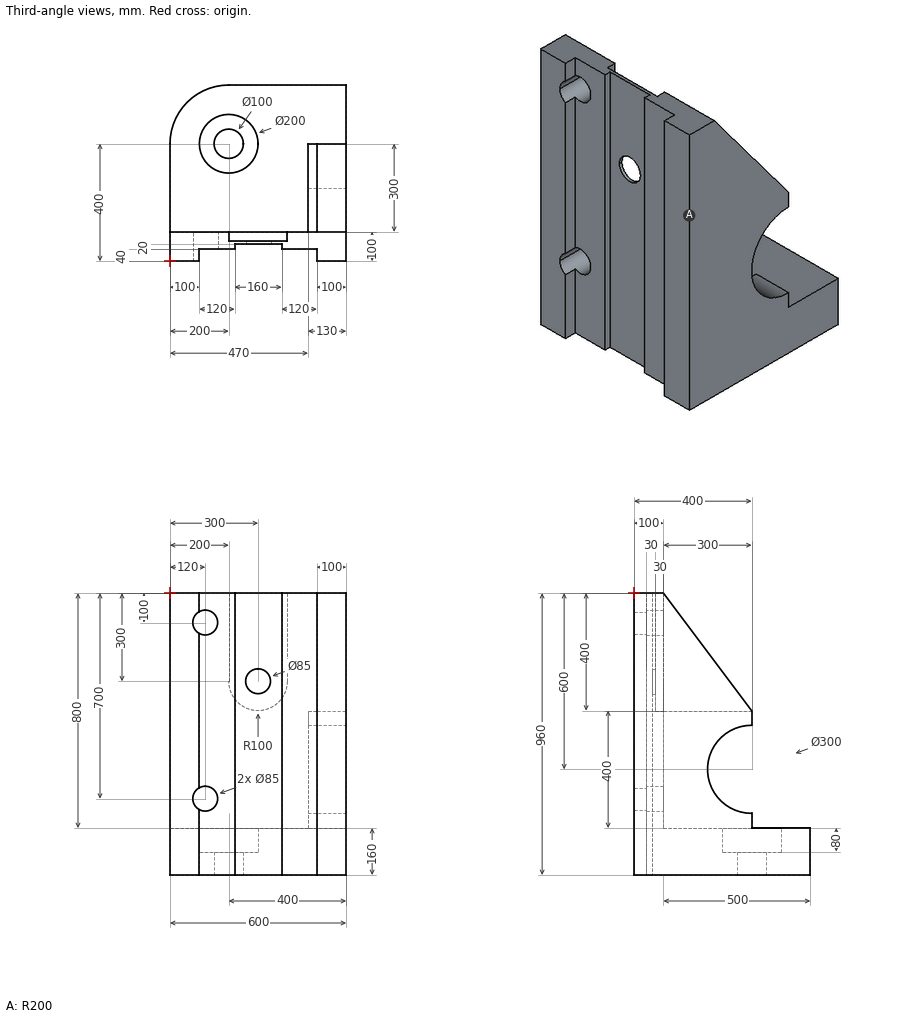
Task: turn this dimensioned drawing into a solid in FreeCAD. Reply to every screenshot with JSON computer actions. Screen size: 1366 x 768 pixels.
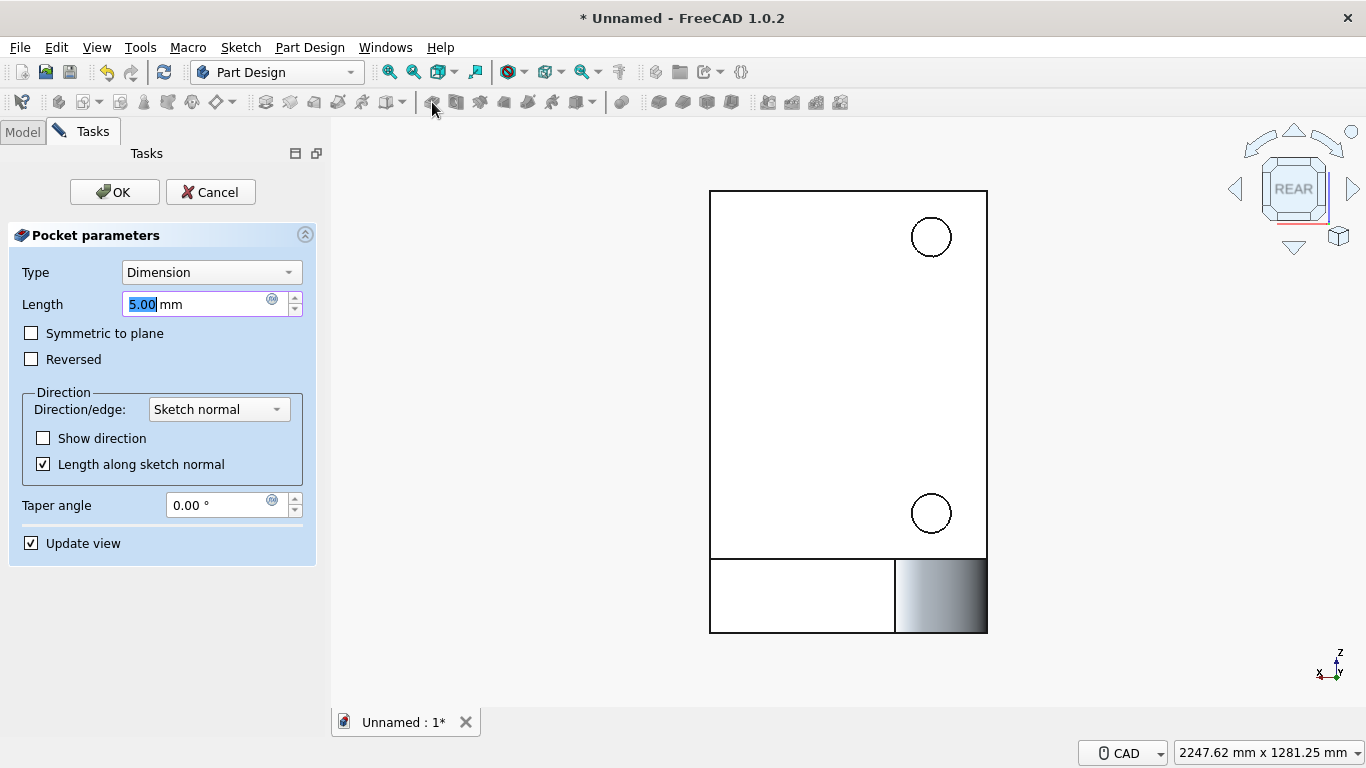
{"action": "left_click", "coordinate": [212, 272]}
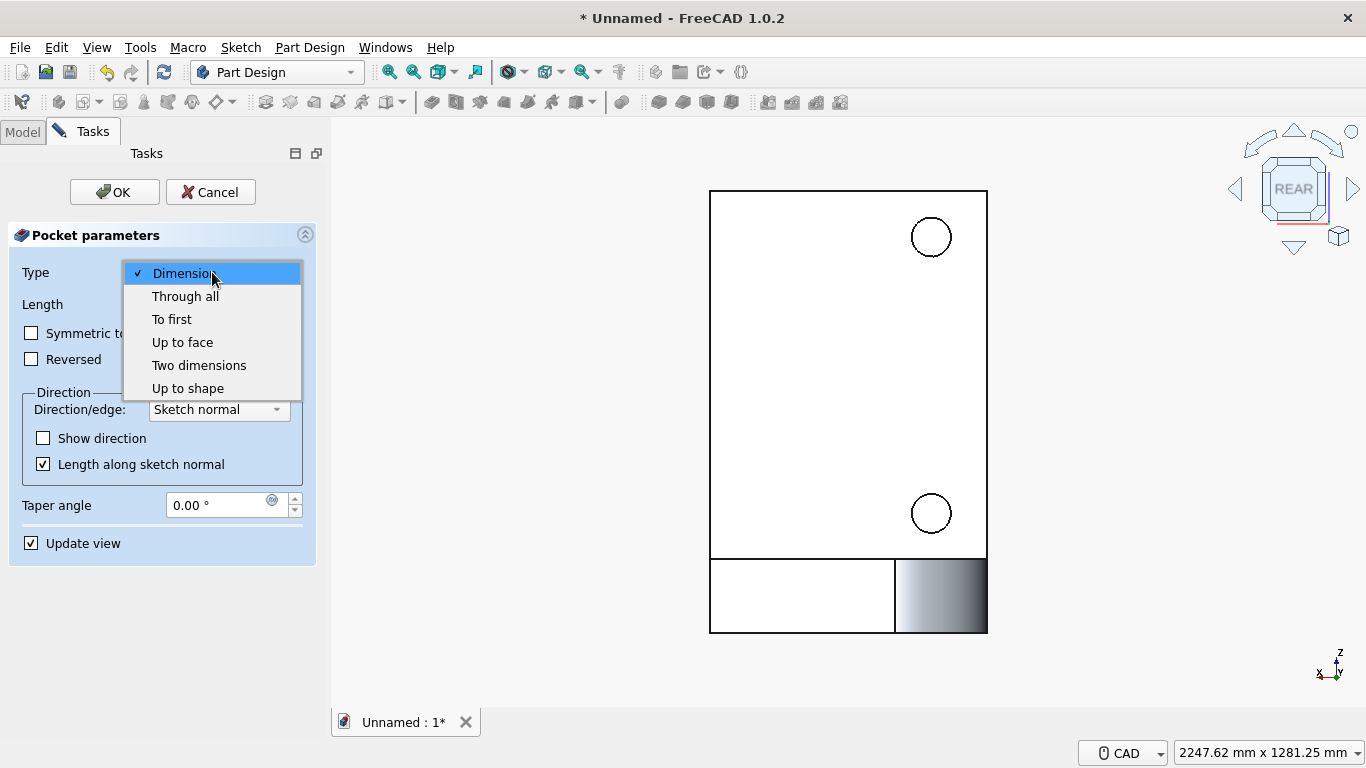
{"action": "left_click", "coordinate": [212, 296]}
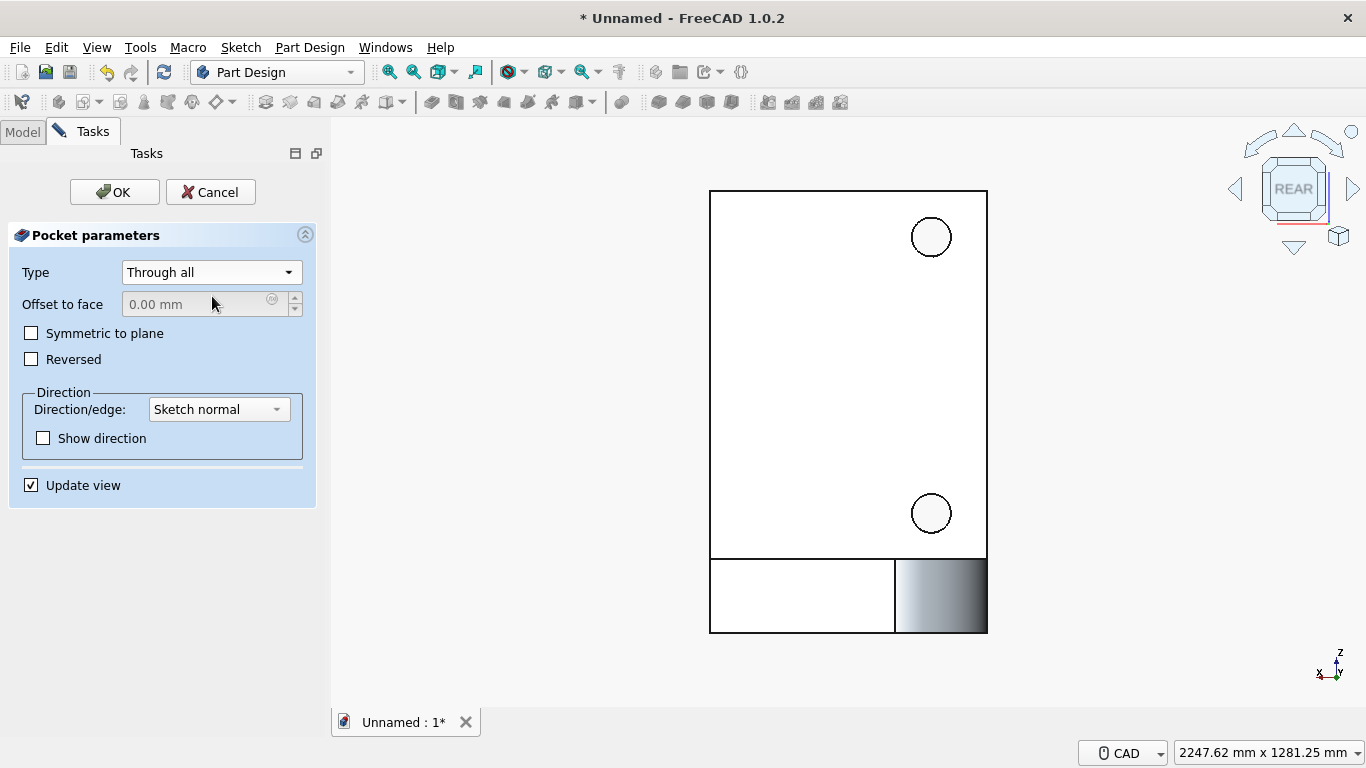
{"action": "left_click", "coordinate": [115, 192]}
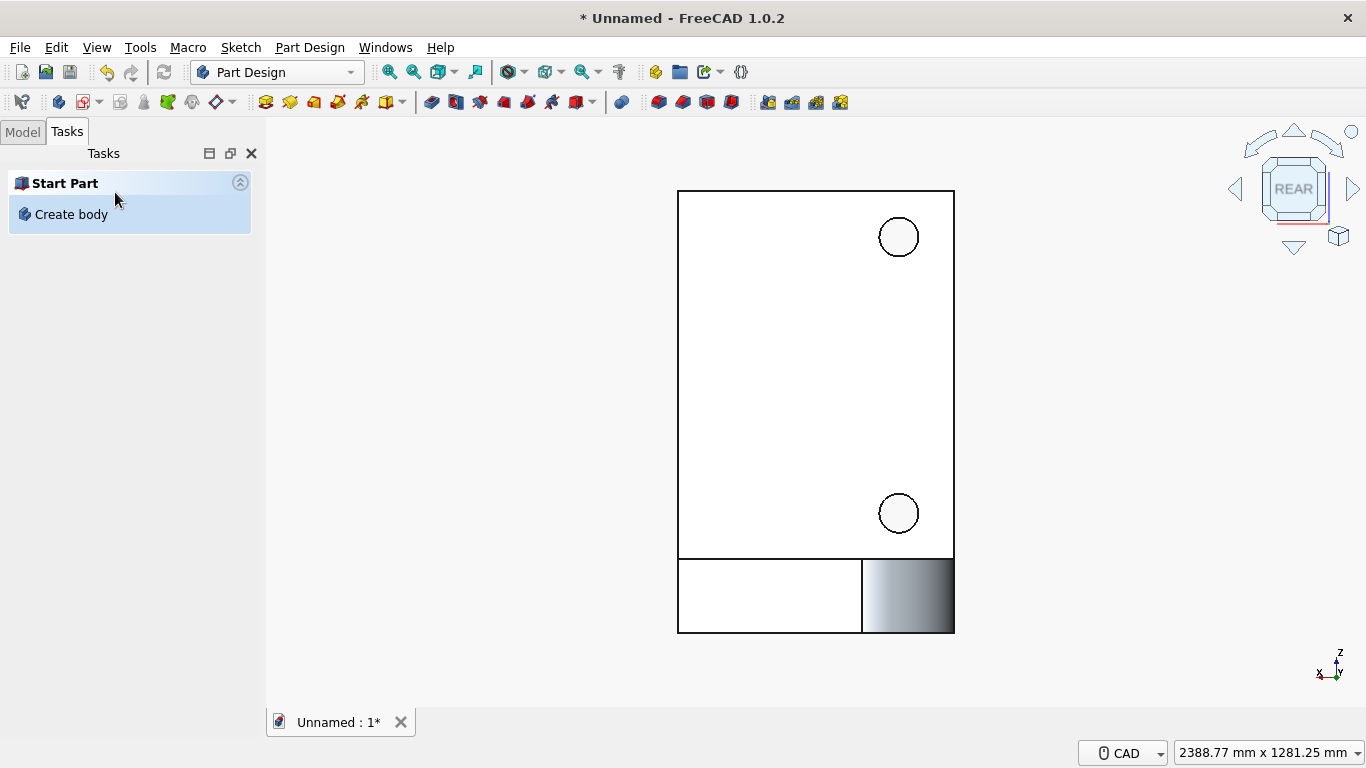
{"action": "left_click", "coordinate": [816, 374]}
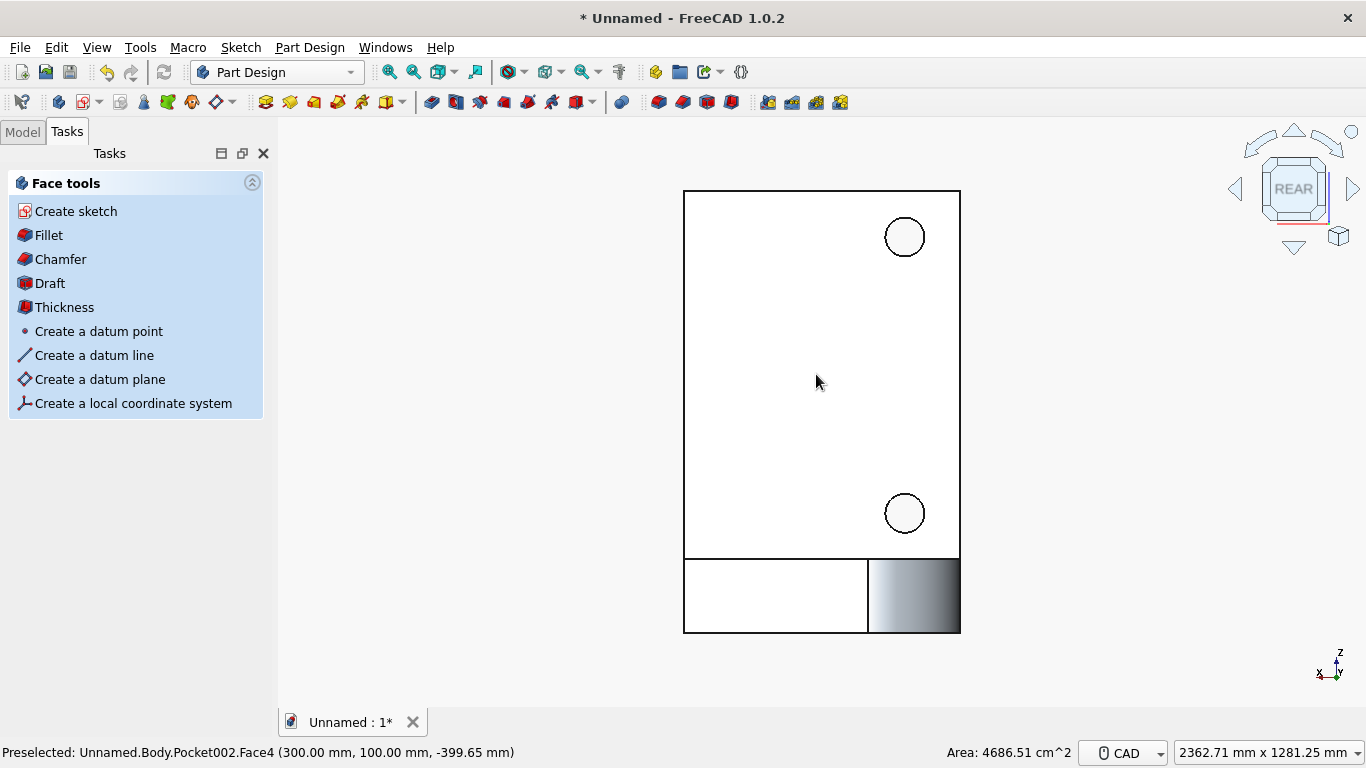
{"action": "left_click", "coordinate": [84, 102]}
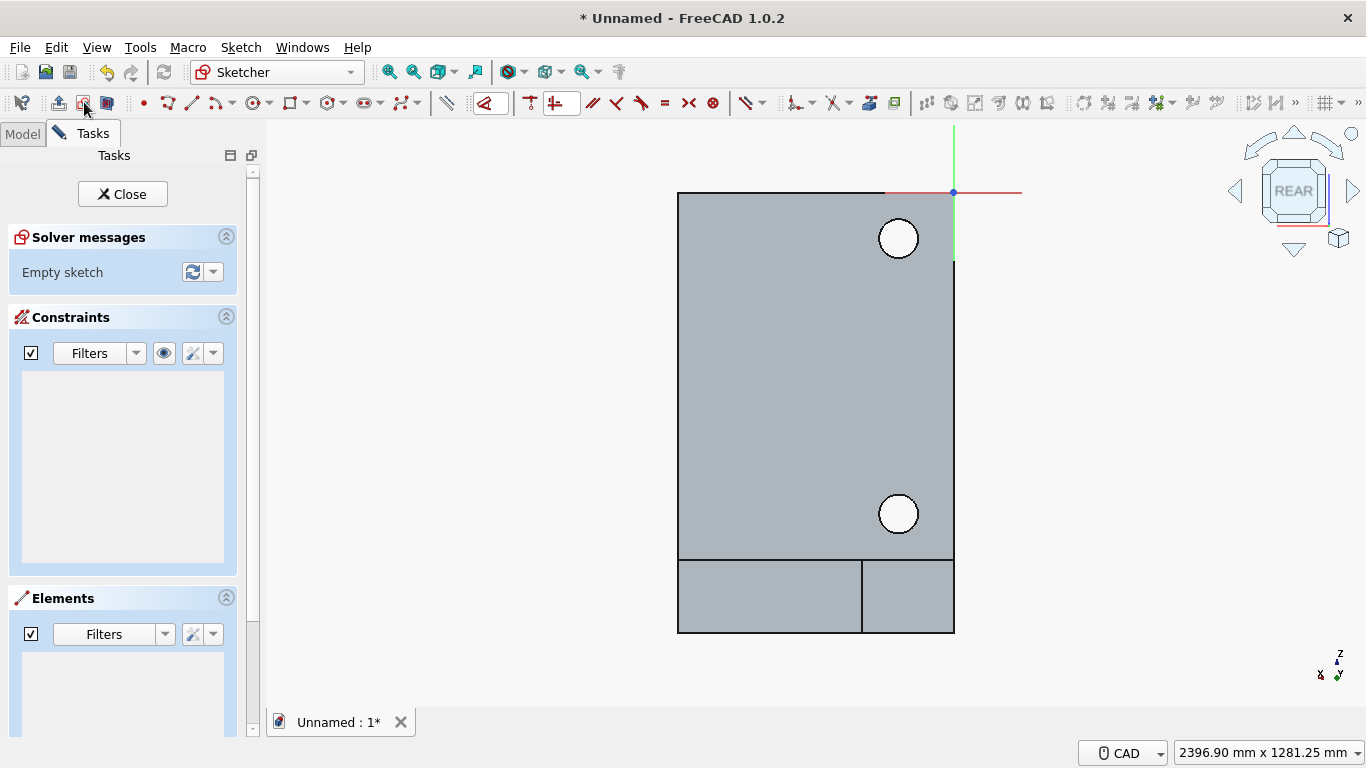
{"action": "scroll", "coordinate": [955, 180], "scroll_direction": "up", "scroll_amount": 4}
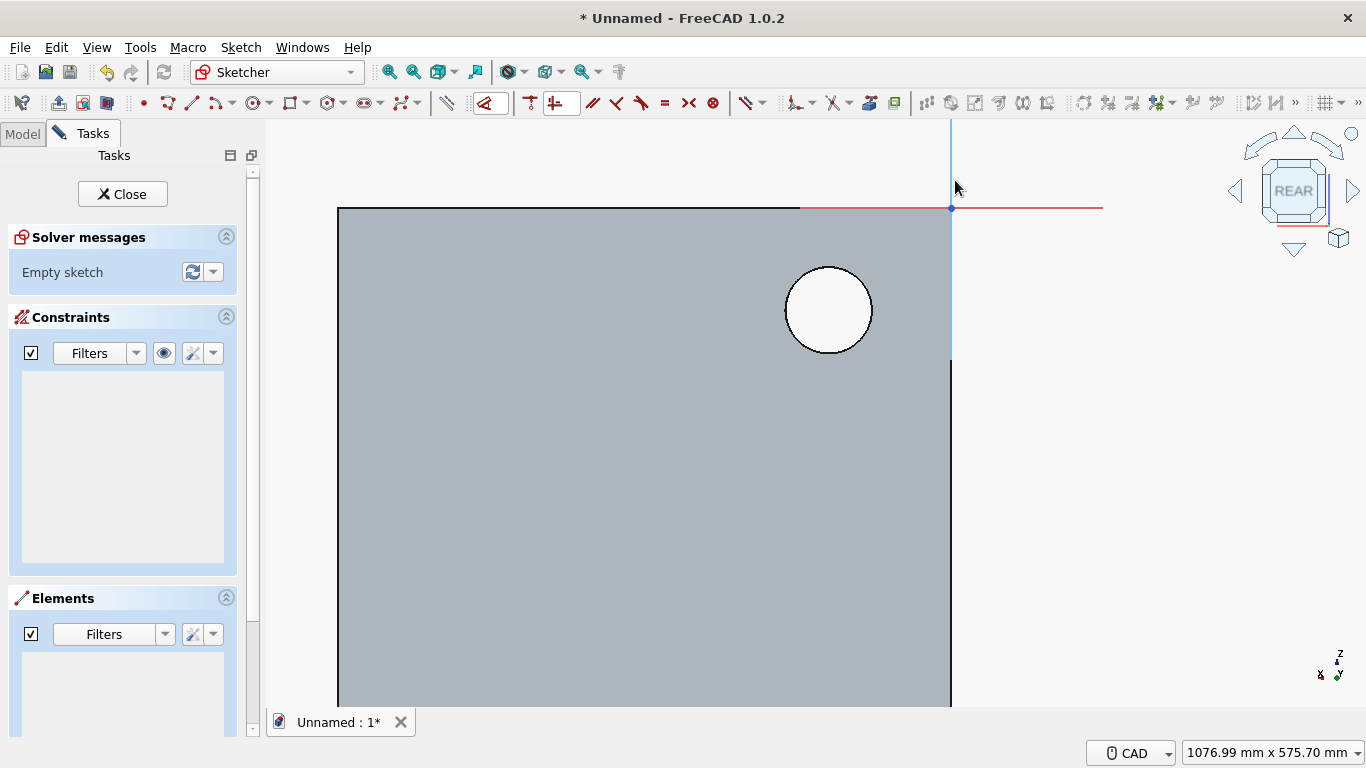
{"action": "left_click", "coordinate": [168, 104]}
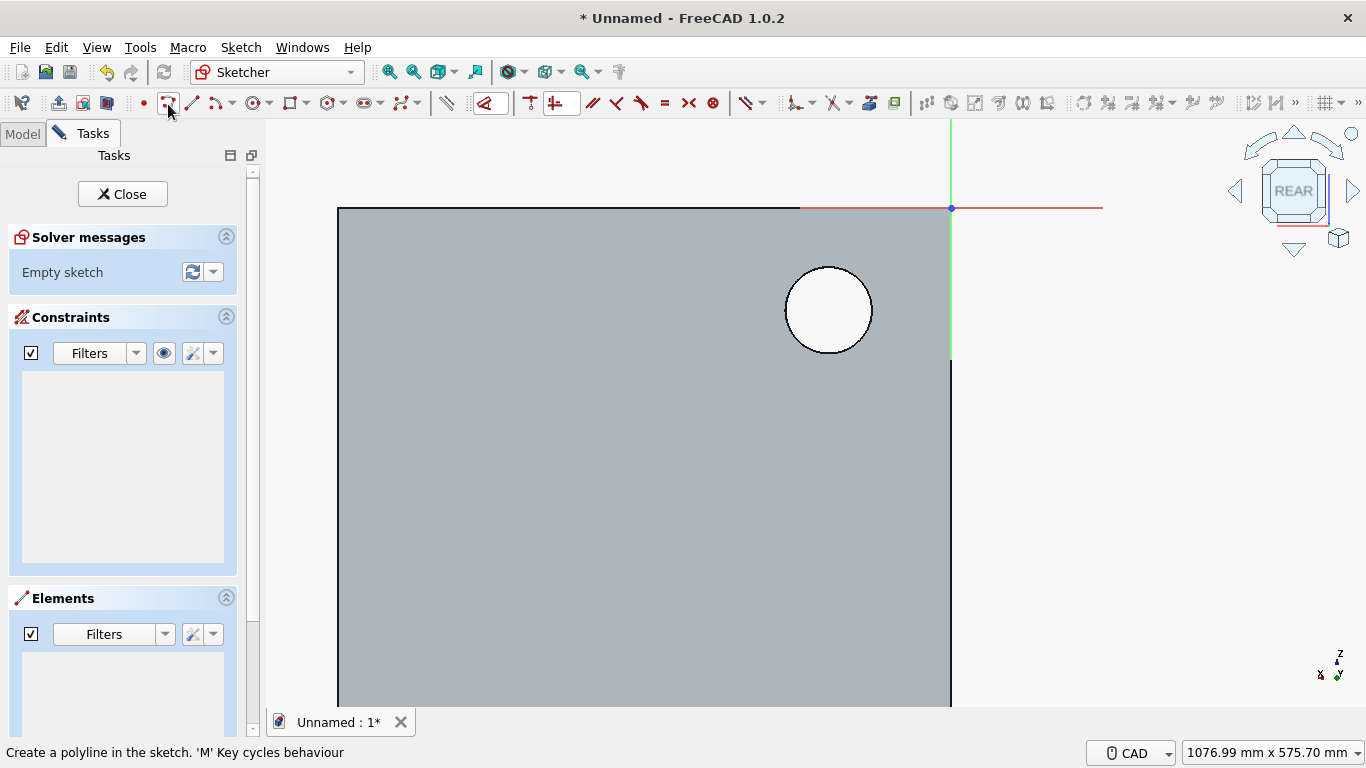
{"action": "left_click", "coordinate": [747, 515]}
{"action": "left_click", "coordinate": [747, 208]}
{"action": "left_click", "coordinate": [543, 217]}
{"action": "left_click", "coordinate": [543, 515]}
{"action": "right_click", "coordinate": [543, 515]}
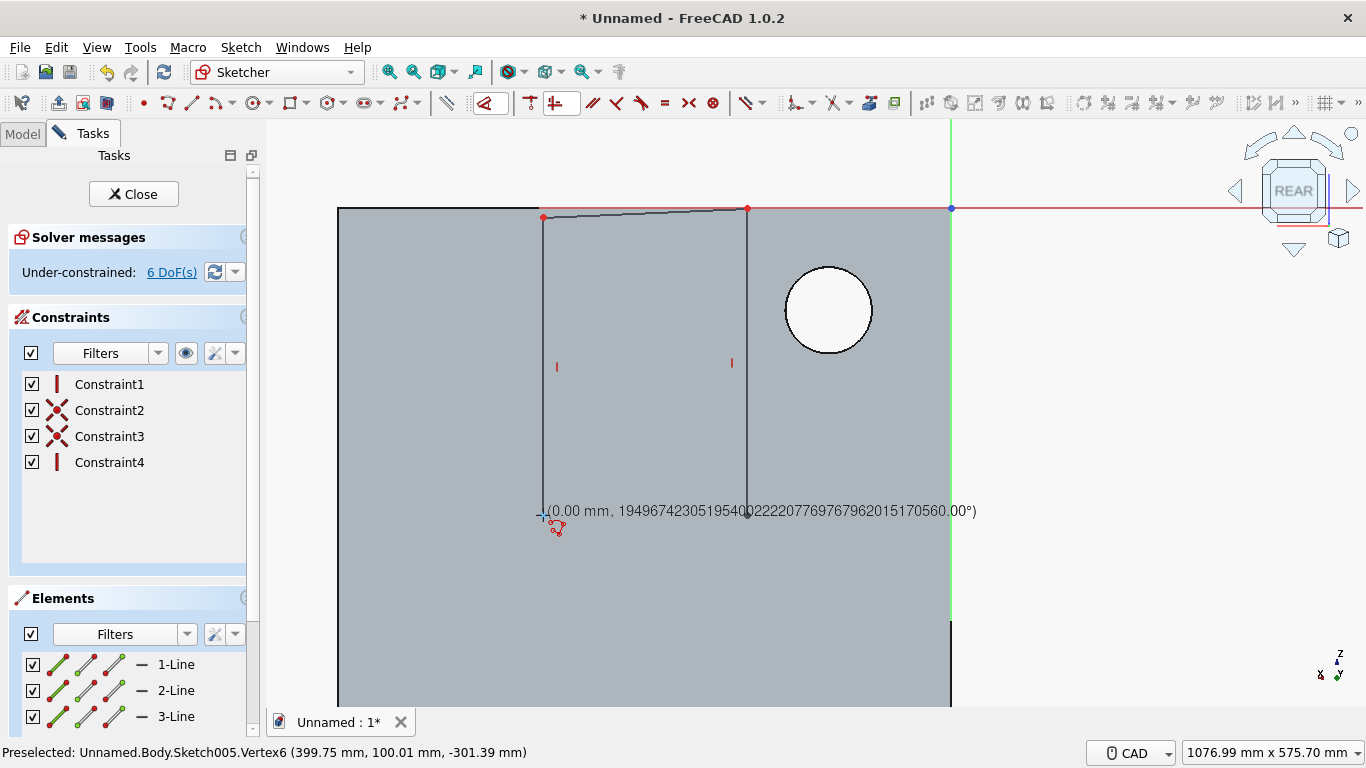
{"action": "left_click", "coordinate": [234, 104]}